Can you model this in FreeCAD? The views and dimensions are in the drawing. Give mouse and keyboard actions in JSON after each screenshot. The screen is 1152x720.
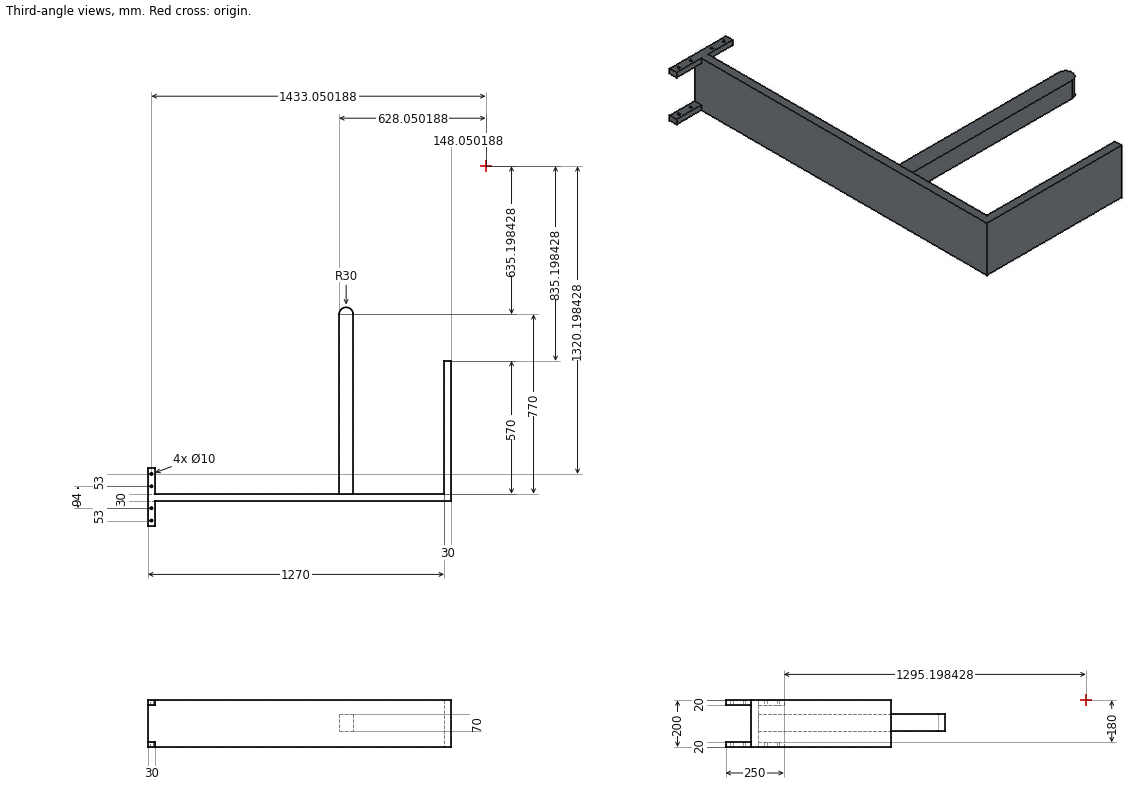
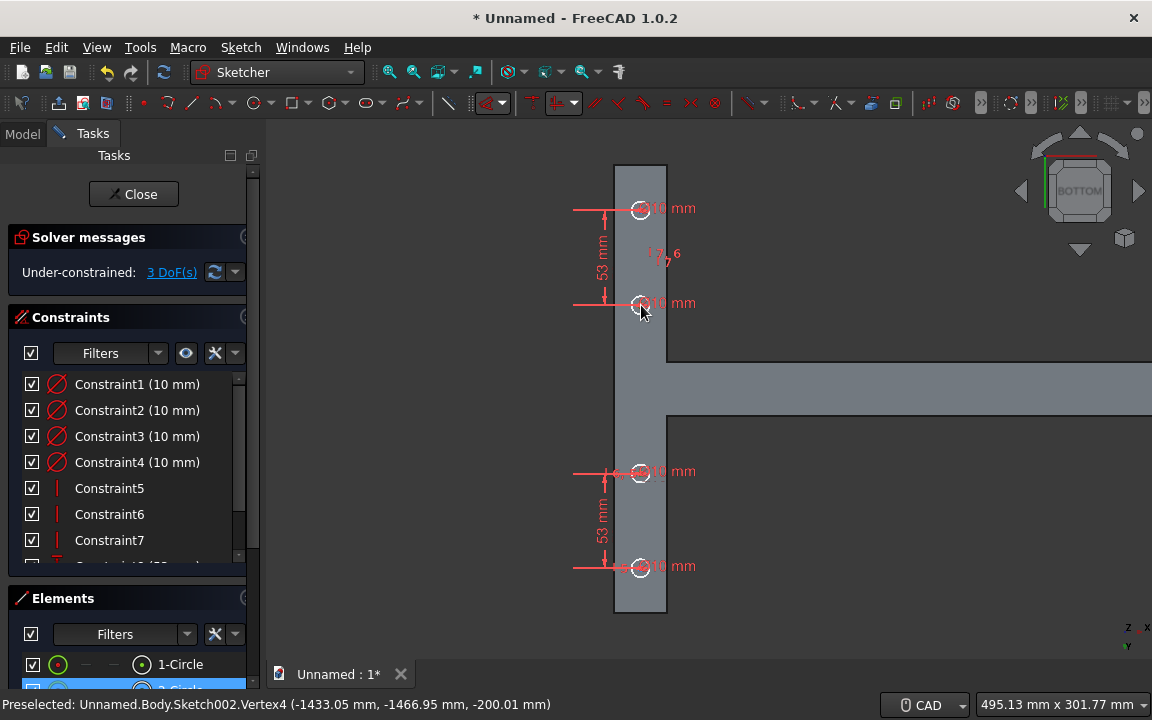
{"action": "left_click", "coordinate": [504, 104]}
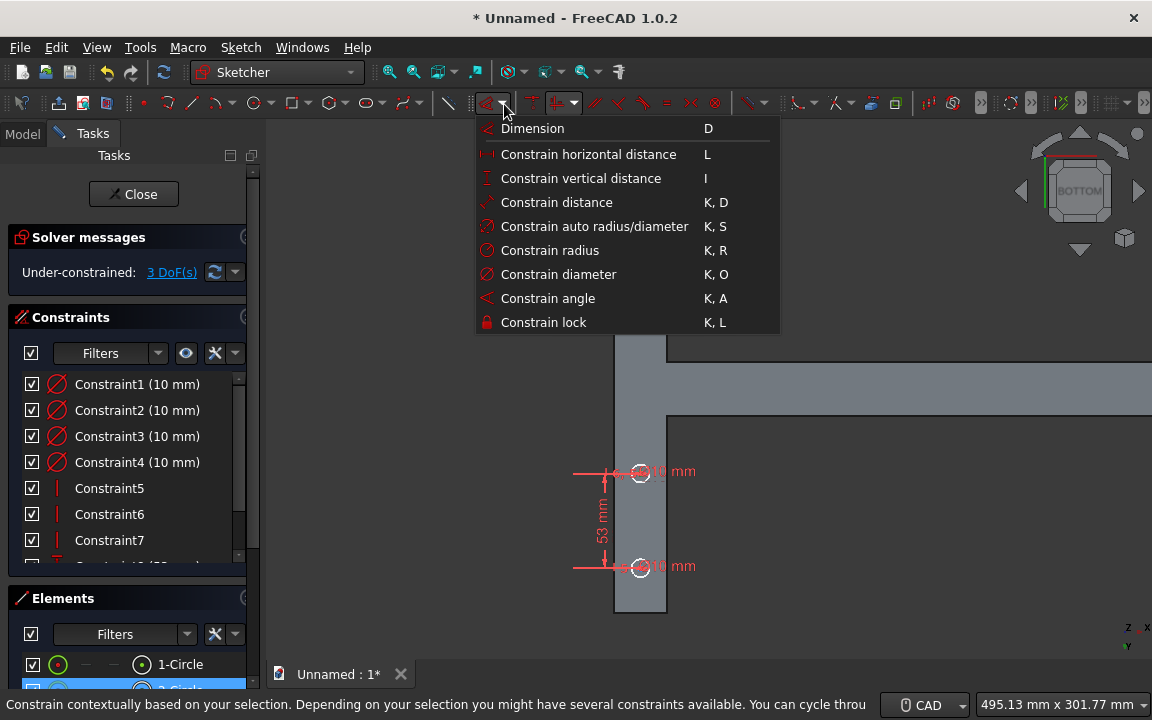
{"action": "left_click", "coordinate": [628, 178]}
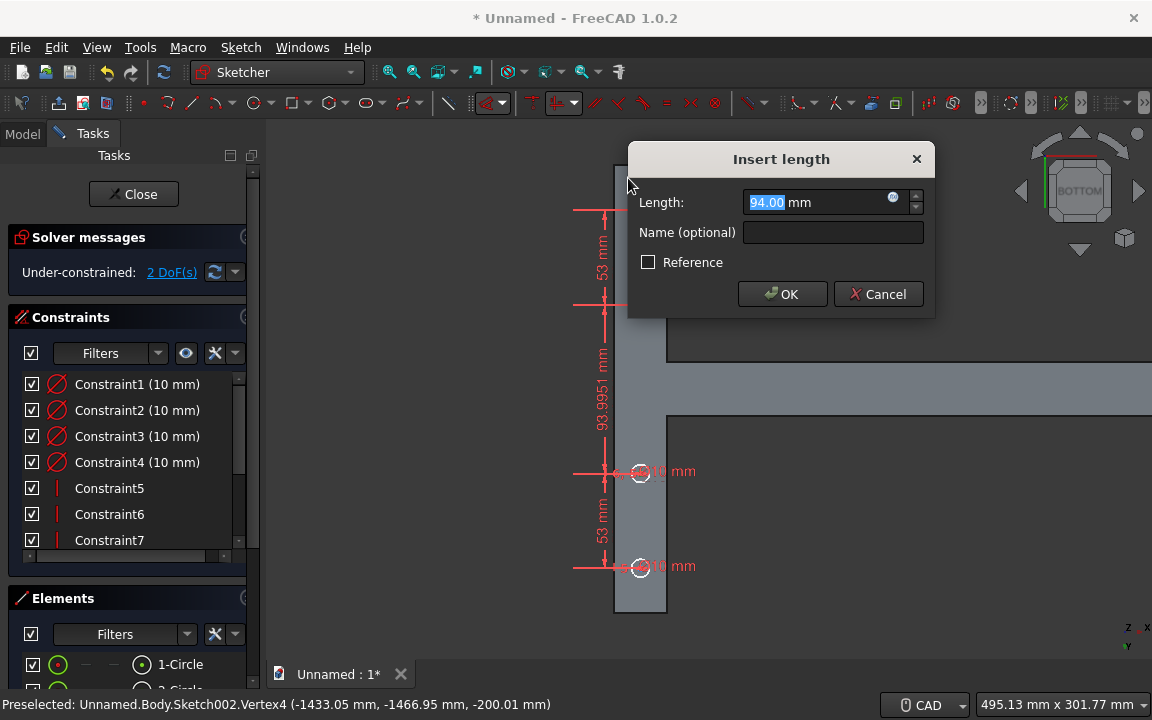
{"action": "type", "text": "94"}
{"action": "key", "text": "Return"}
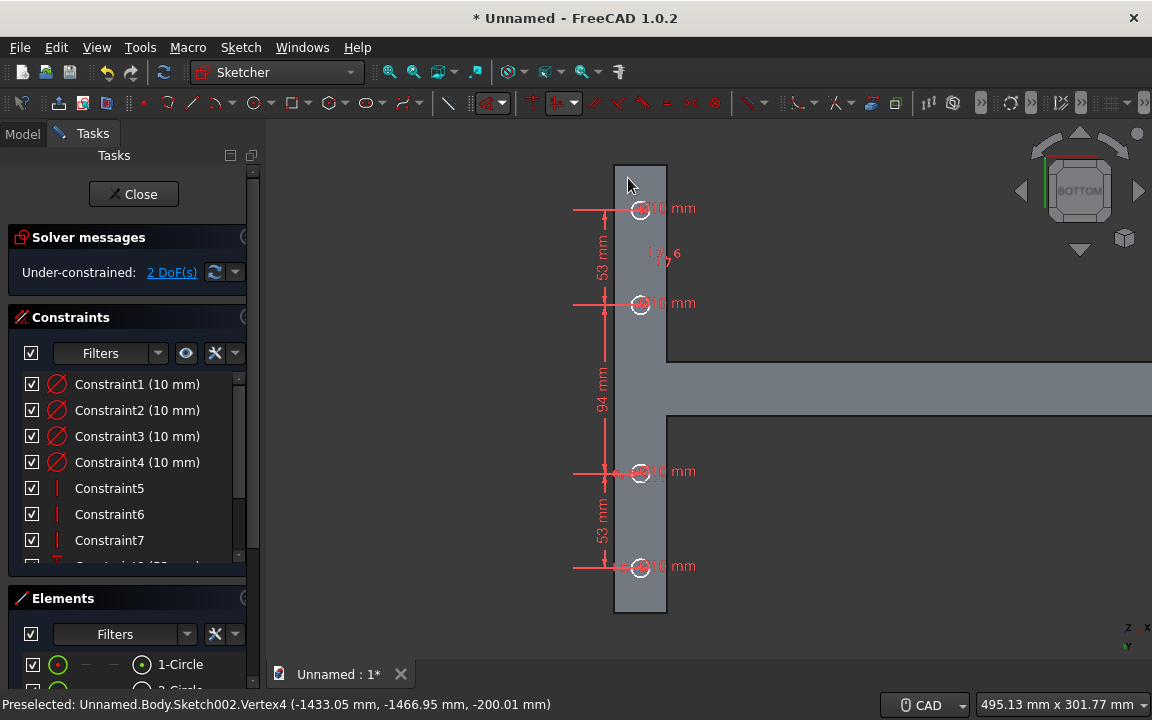
{"action": "left_click", "coordinate": [641, 568]}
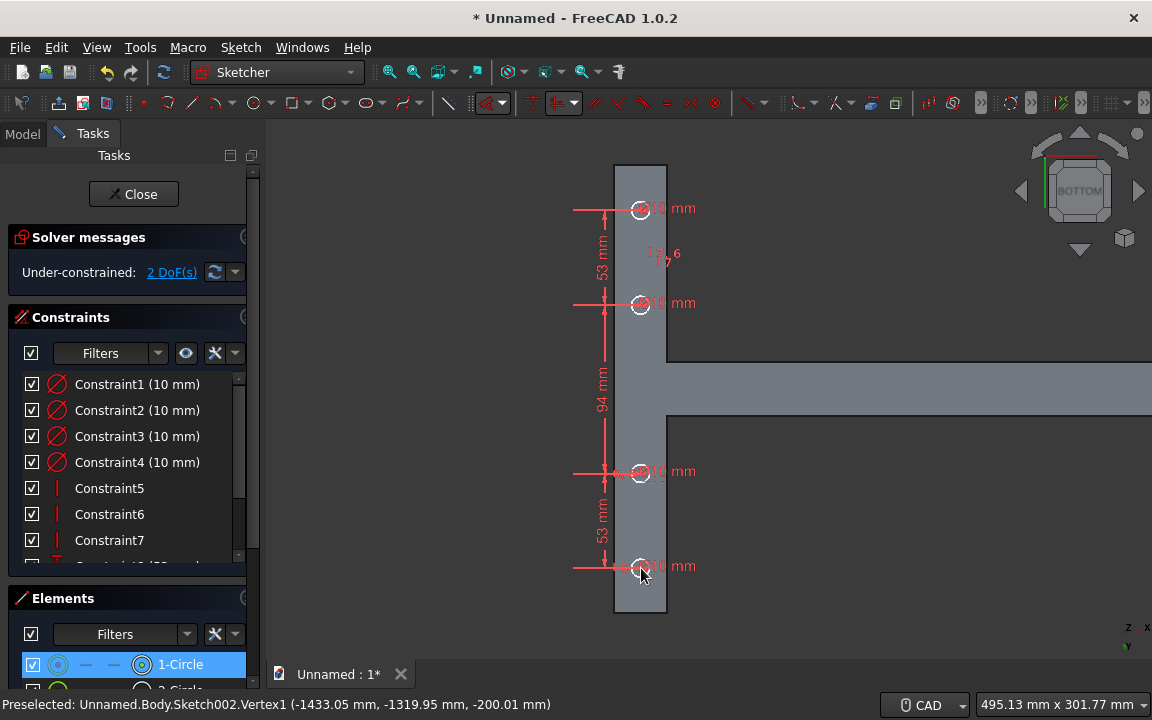
{"action": "left_click", "coordinate": [504, 104]}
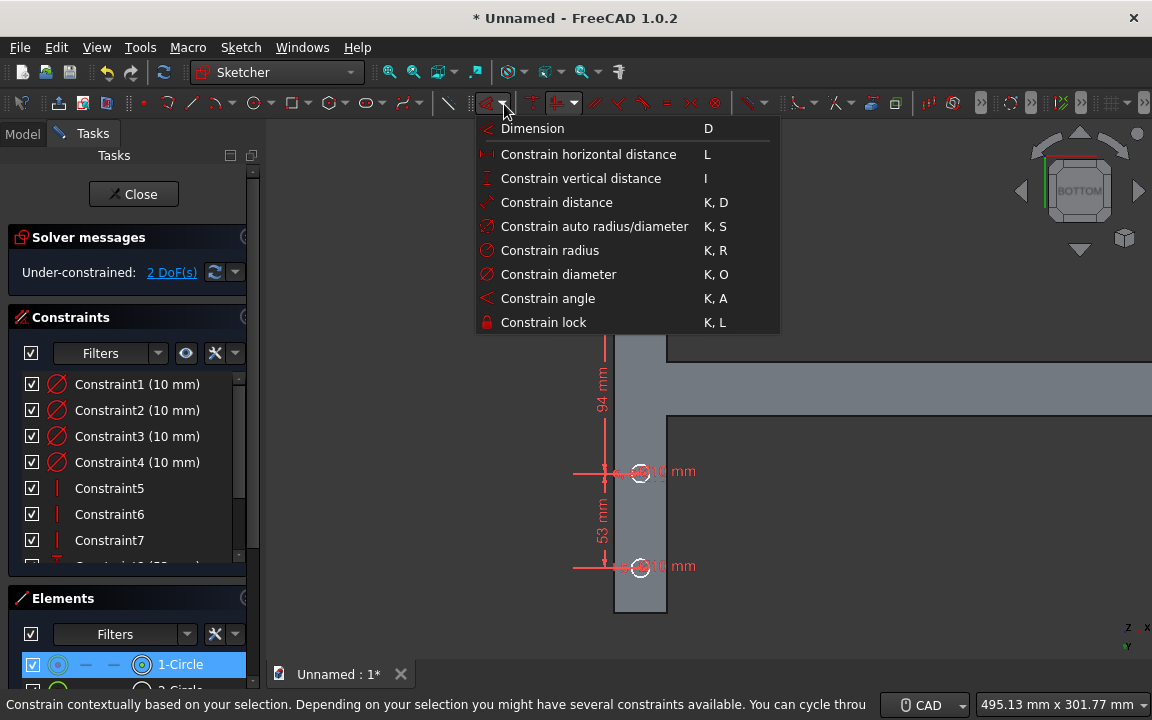
{"action": "left_click", "coordinate": [628, 154]}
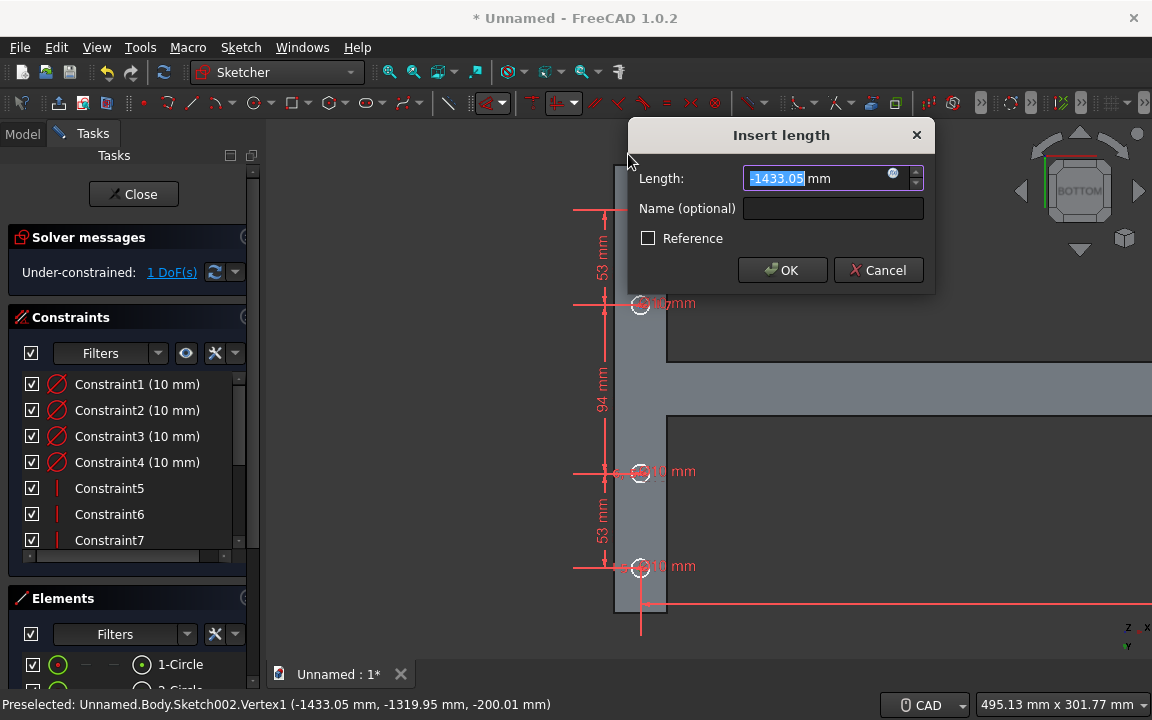
{"action": "type", "text": "-1433.050188"}
{"action": "key", "text": "Return"}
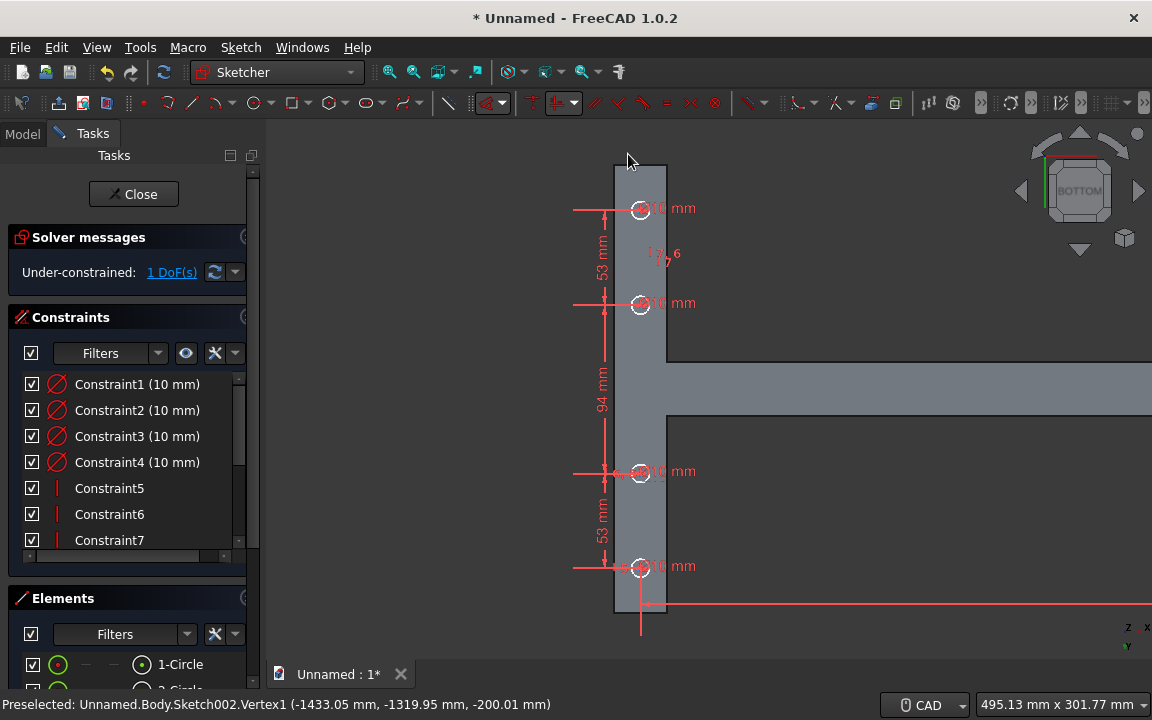
{"action": "left_click", "coordinate": [641, 568]}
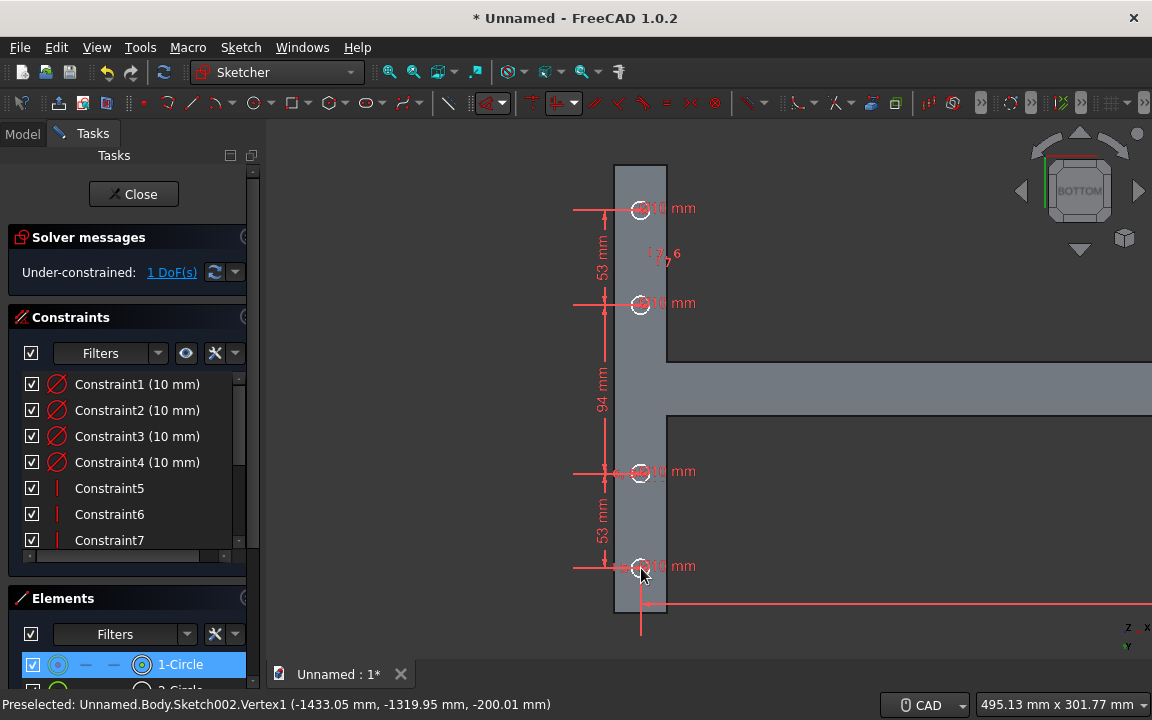
{"action": "left_click", "coordinate": [504, 104]}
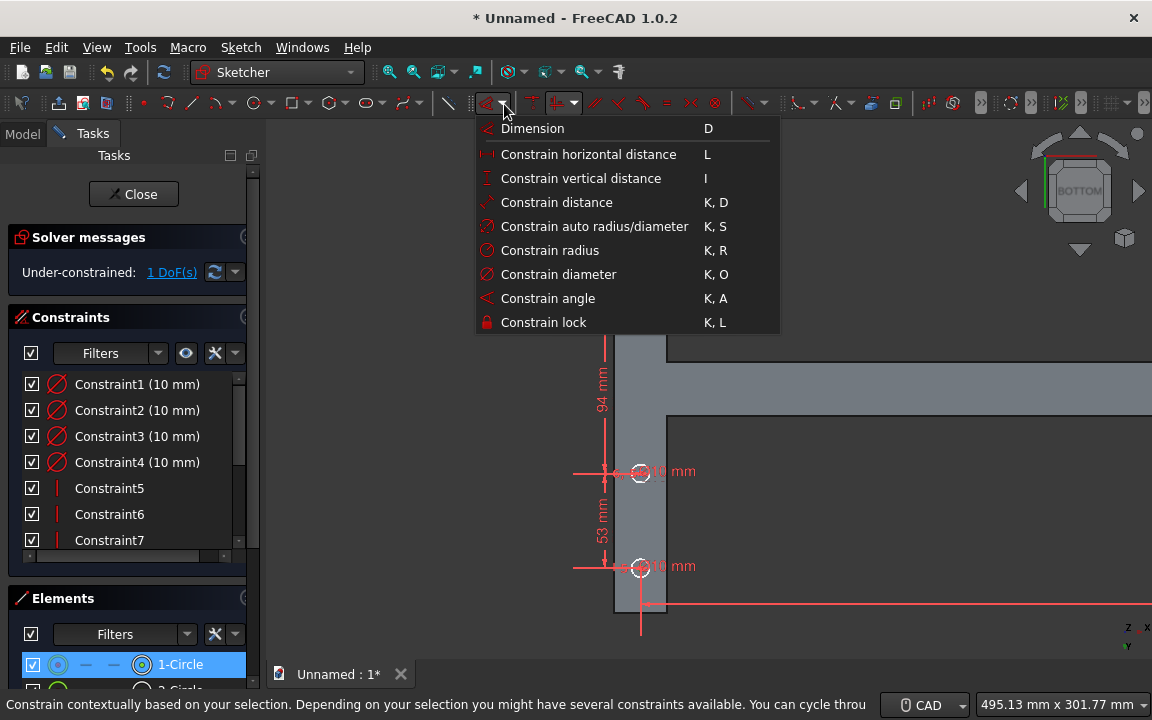
{"action": "left_click", "coordinate": [628, 178]}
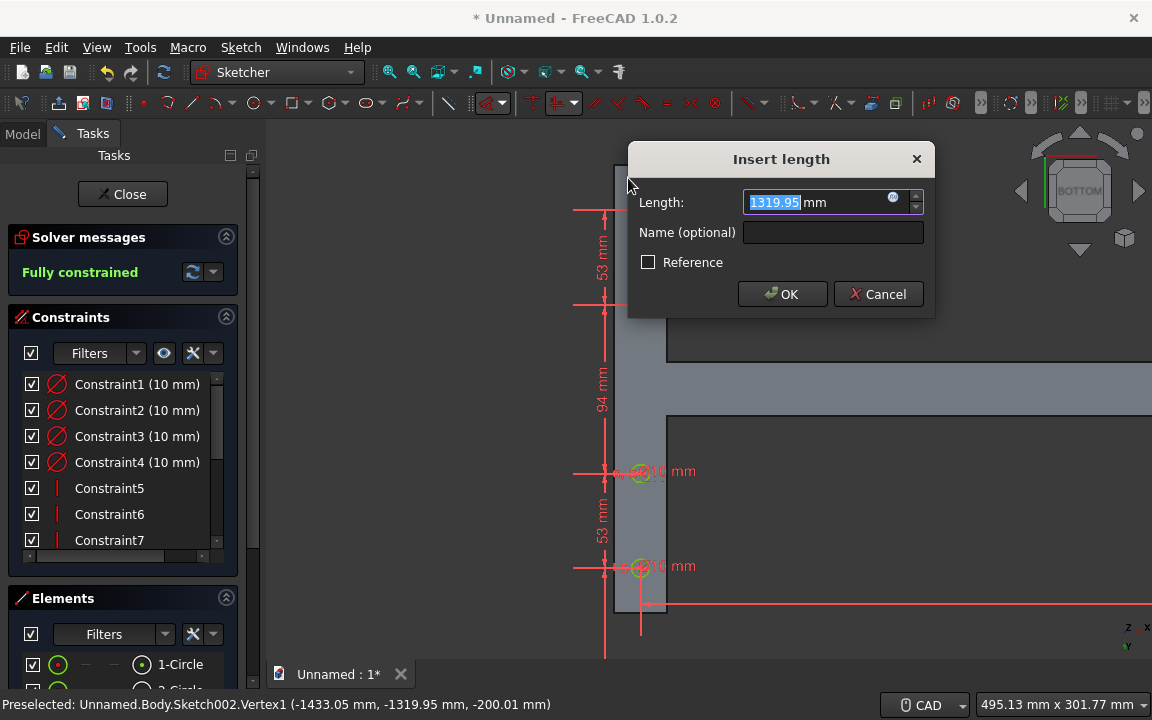
{"action": "type", "text": "1320.198428"}
{"action": "key", "text": "Return"}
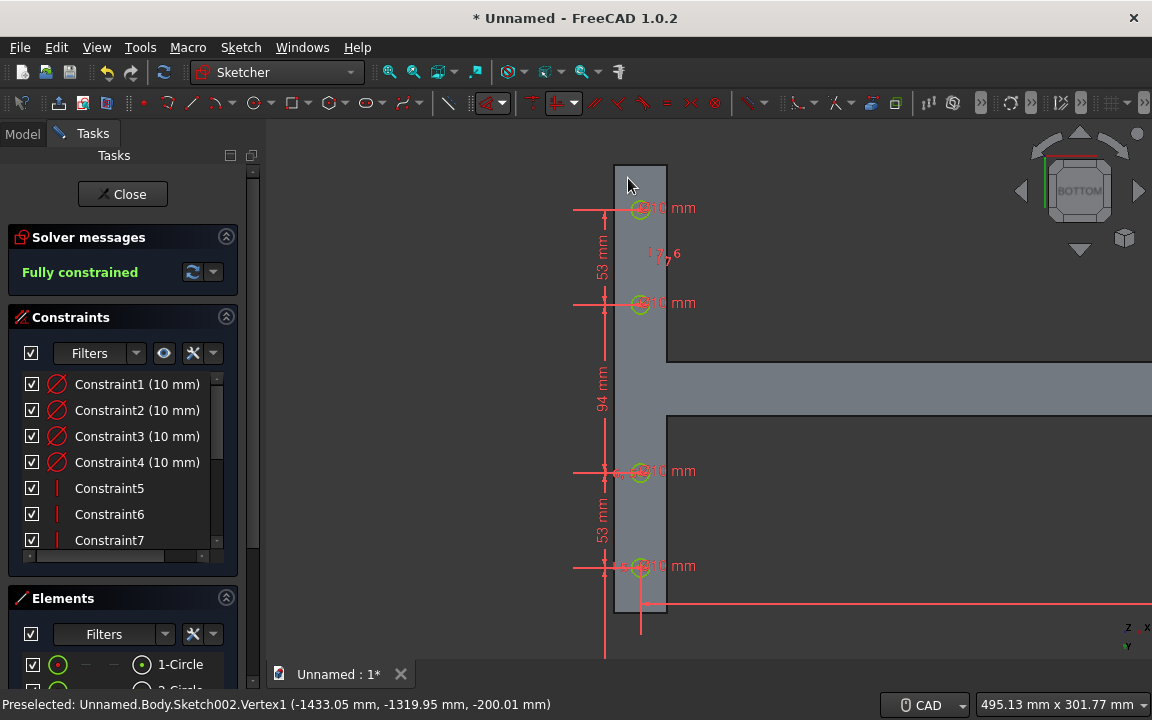
{"action": "left_click", "coordinate": [123, 194]}